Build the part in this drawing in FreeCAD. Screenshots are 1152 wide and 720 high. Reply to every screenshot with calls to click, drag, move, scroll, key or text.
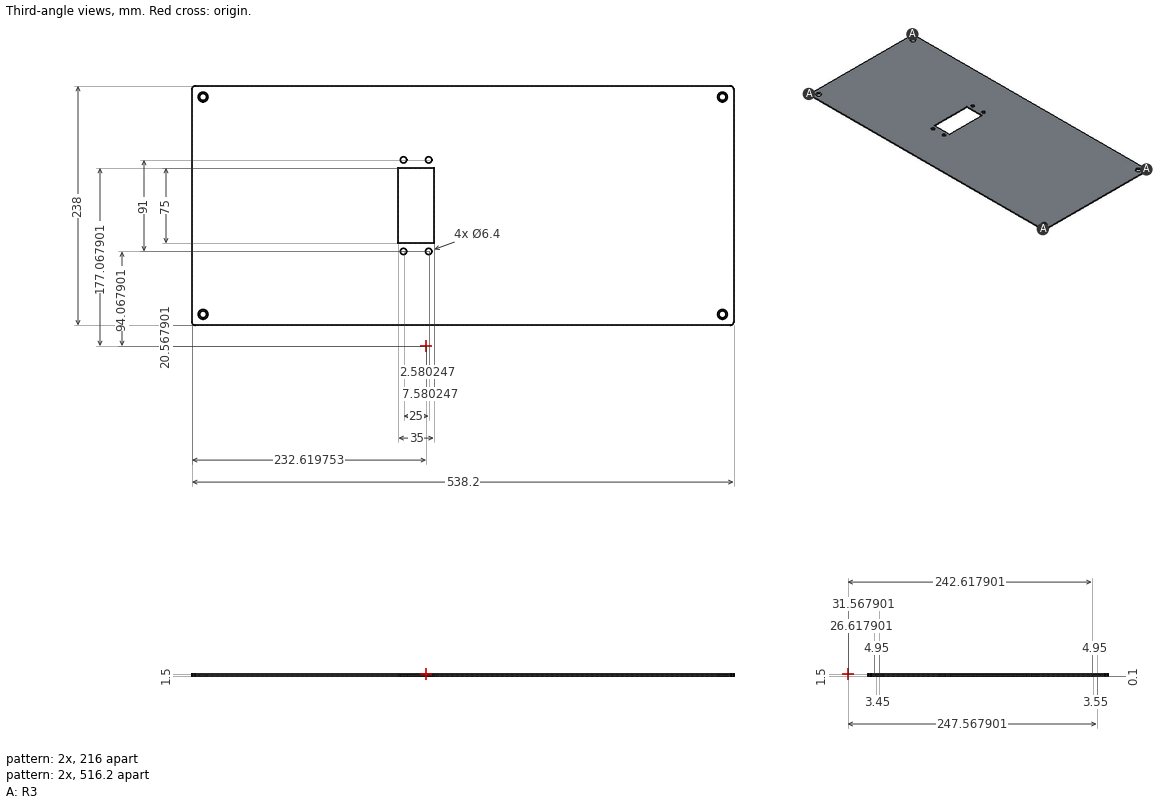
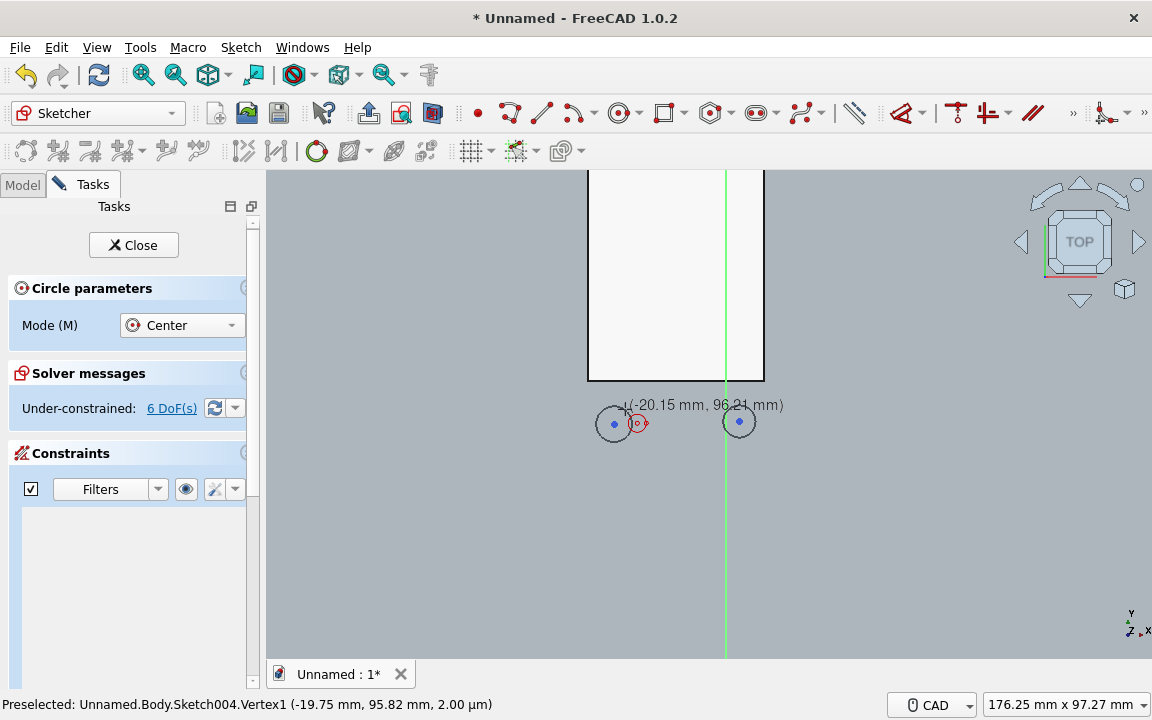
scroll(625, 412, down, 6)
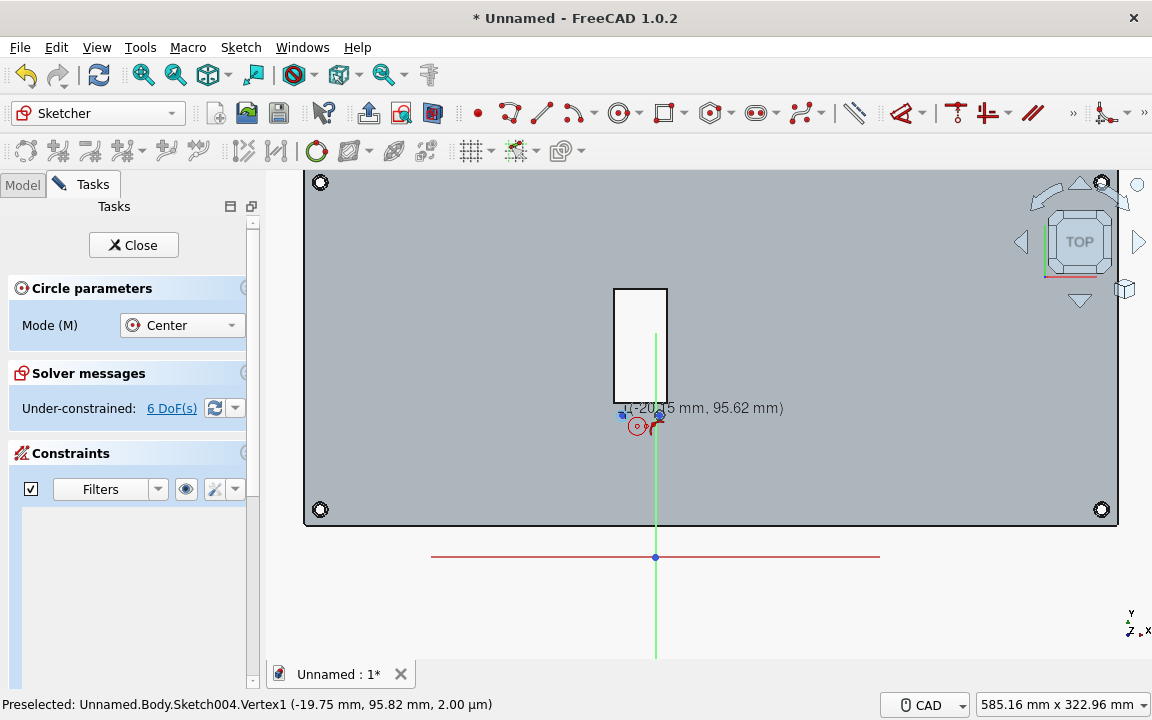
scroll(660, 277, up, 8)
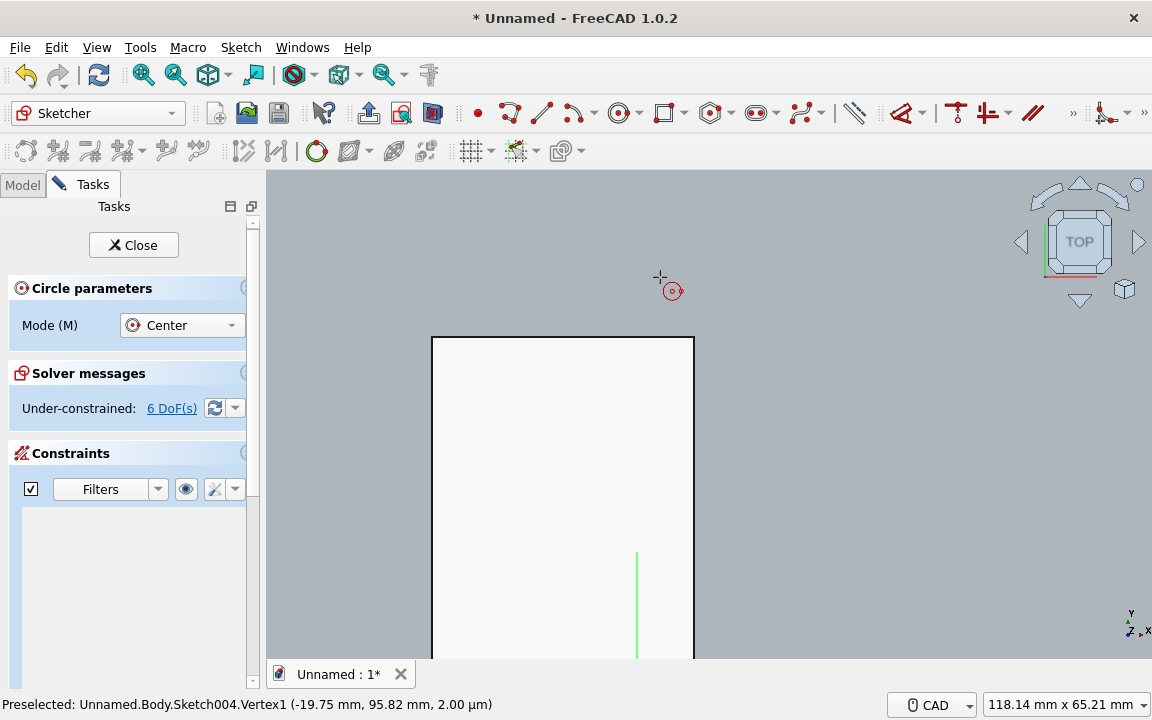
click(657, 277)
click(674, 260)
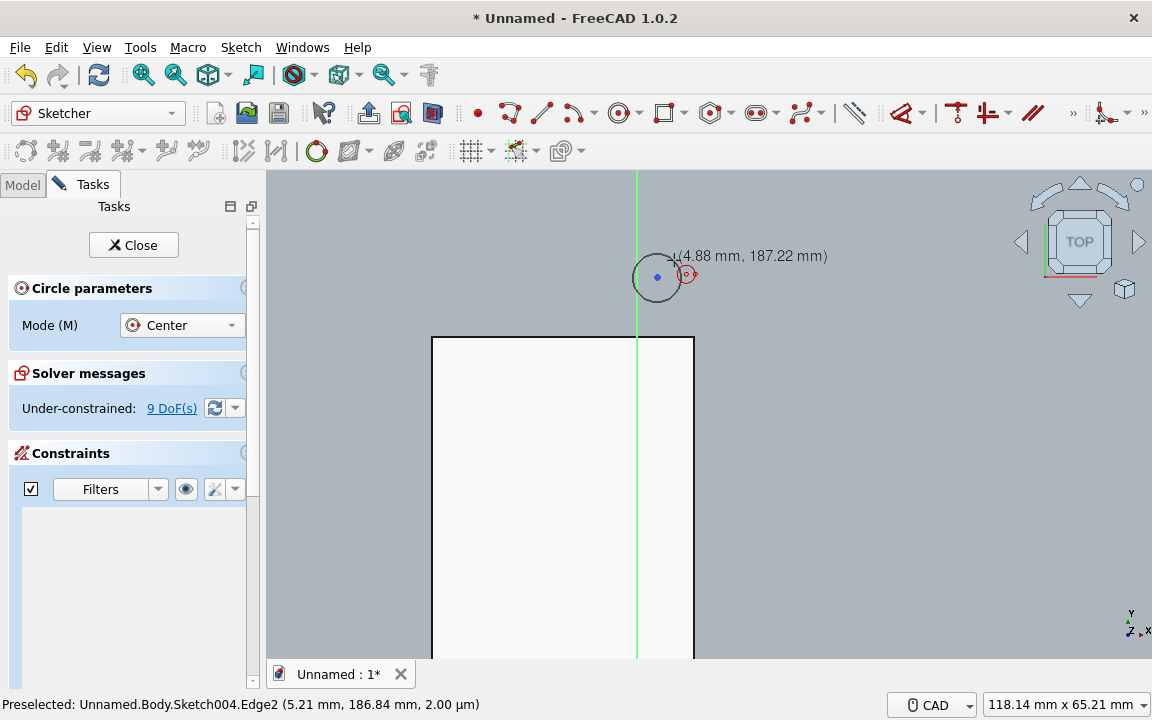
scroll(660, 277, down, 8)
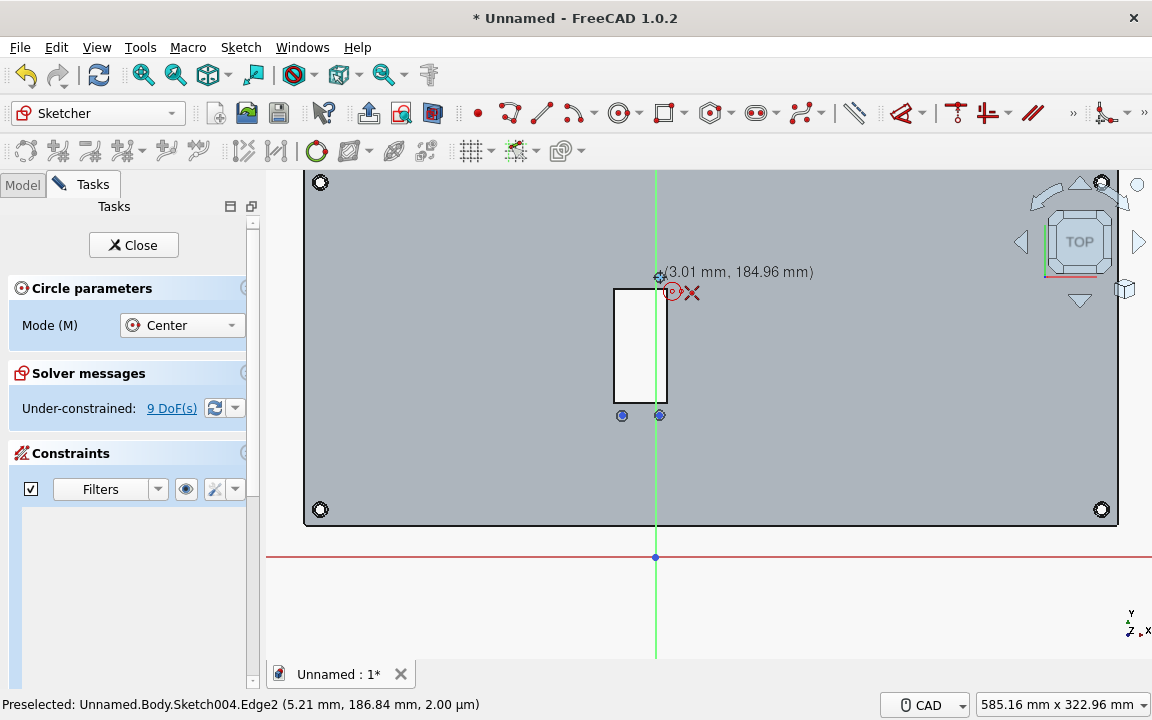
click(622, 277)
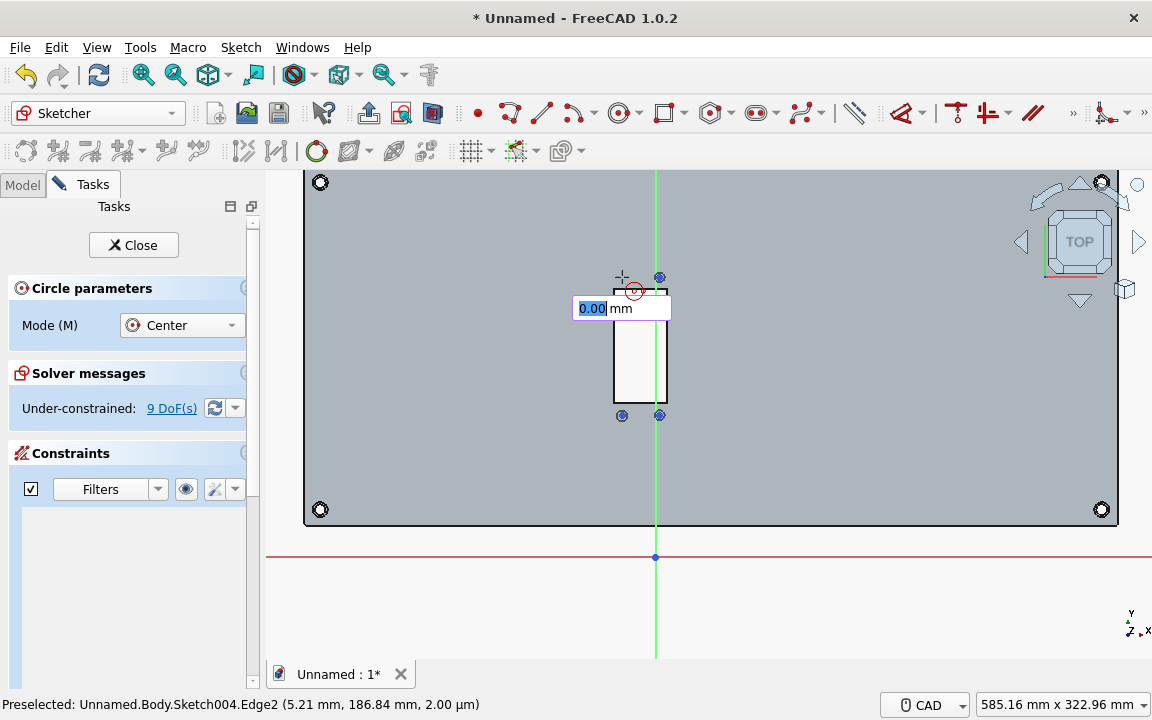
scroll(625, 274, up, 6)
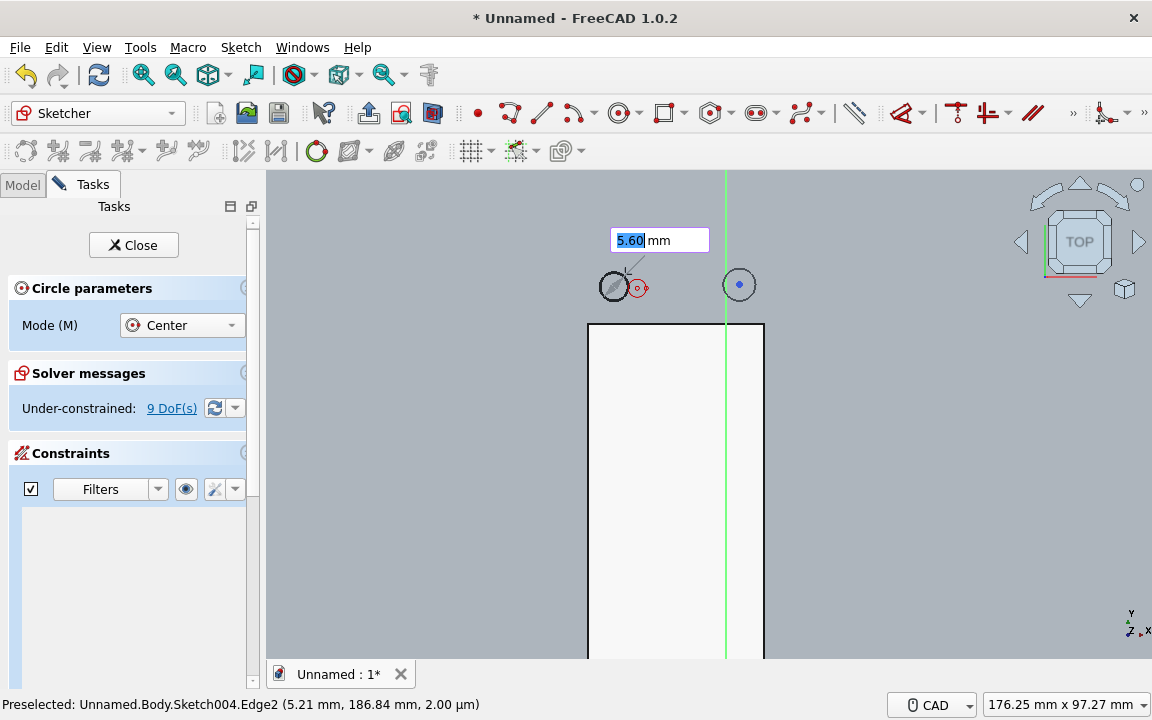
click(625, 273)
key(Escape)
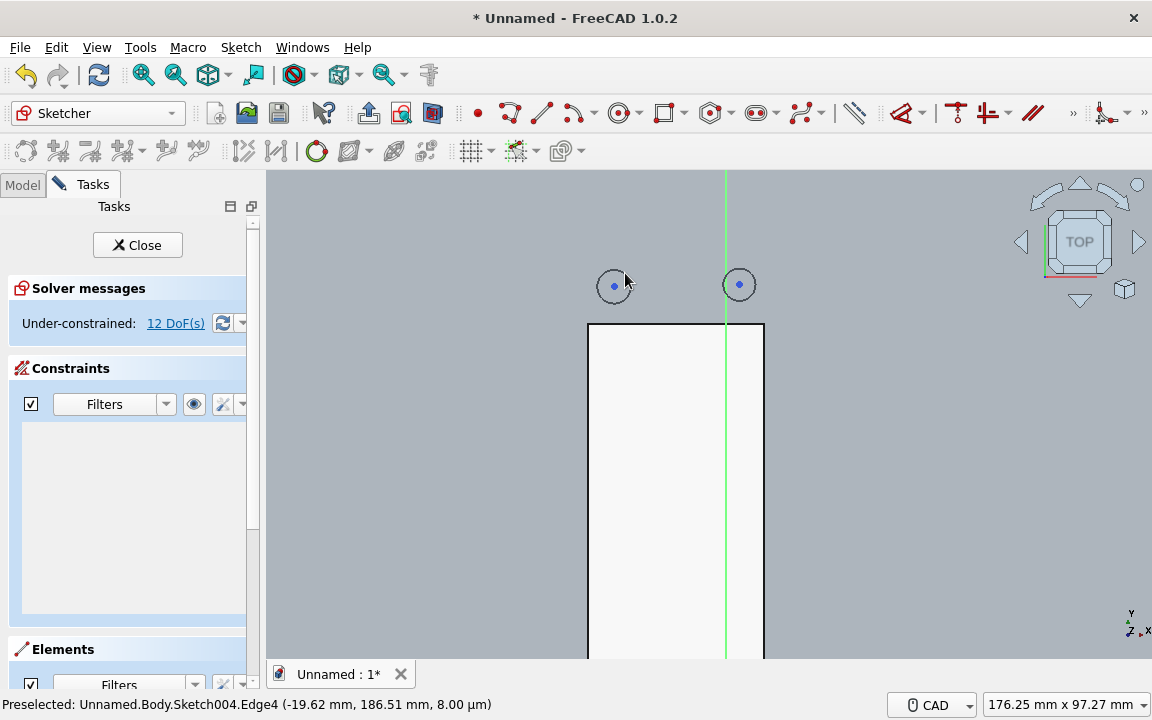
scroll(625, 274, down, 6)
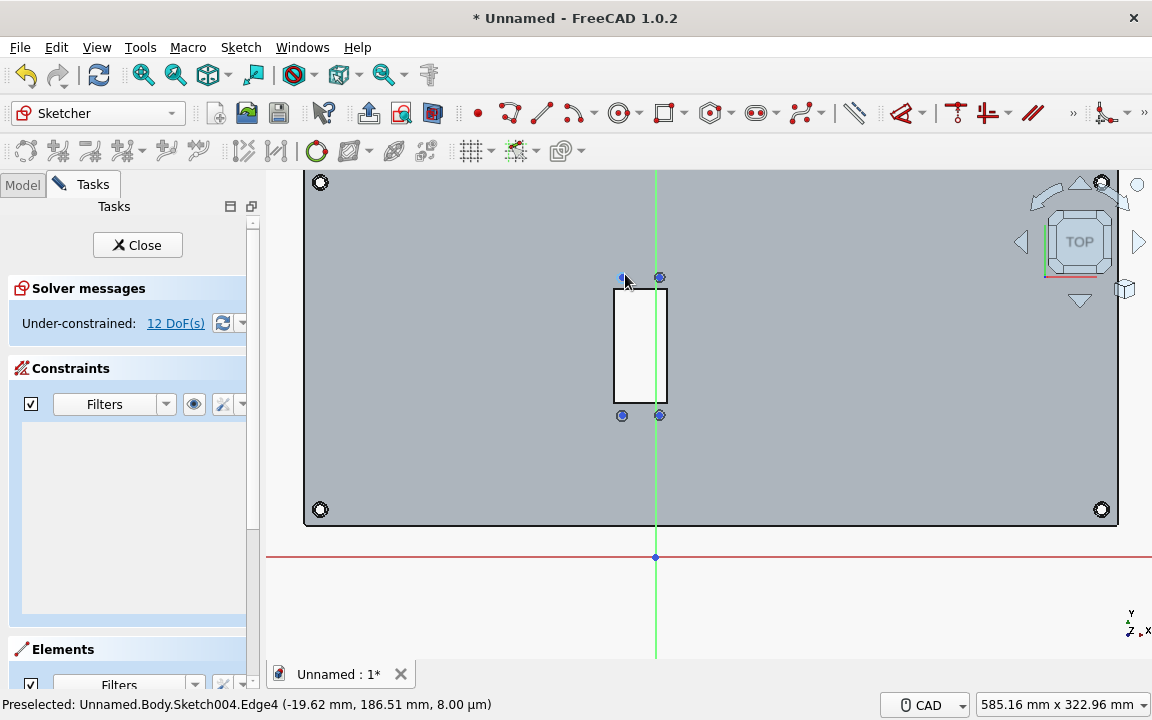
scroll(663, 412, up, 6)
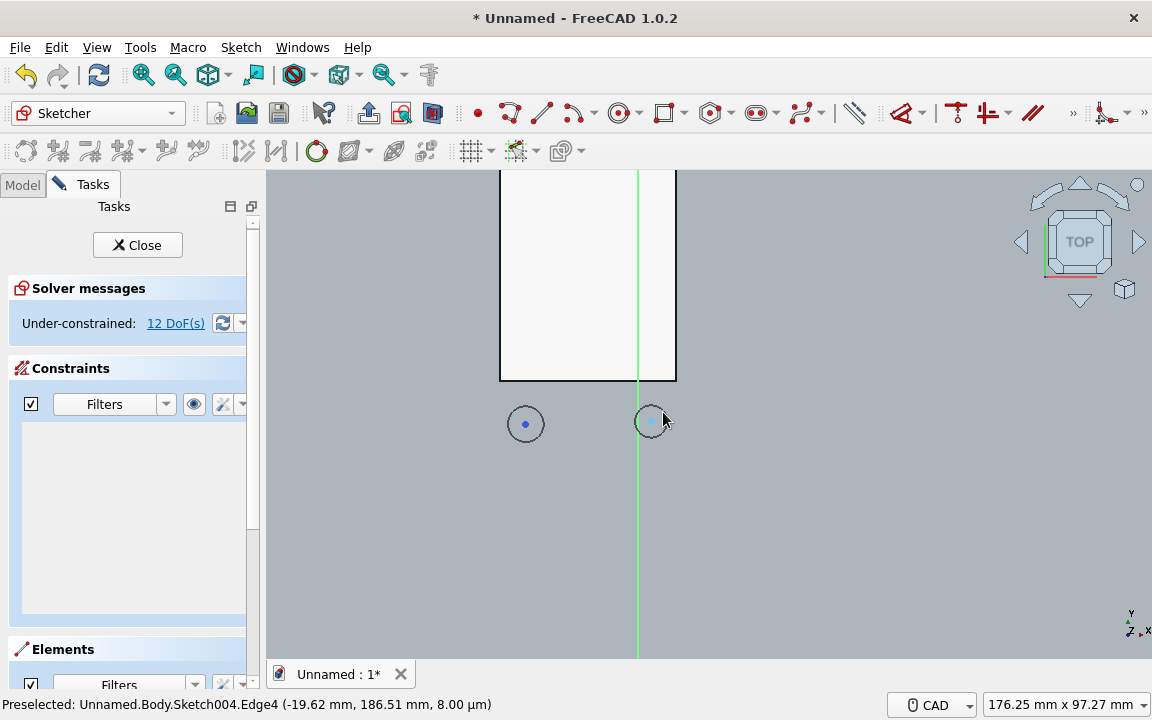
click(663, 410)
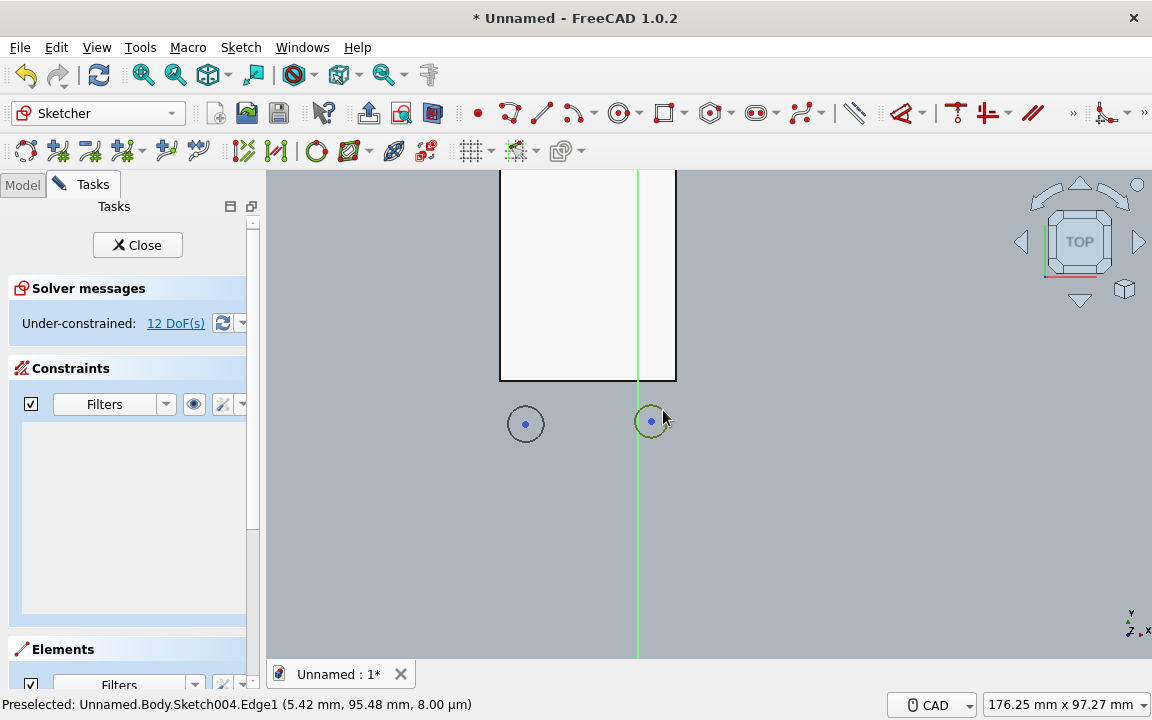
click(538, 411)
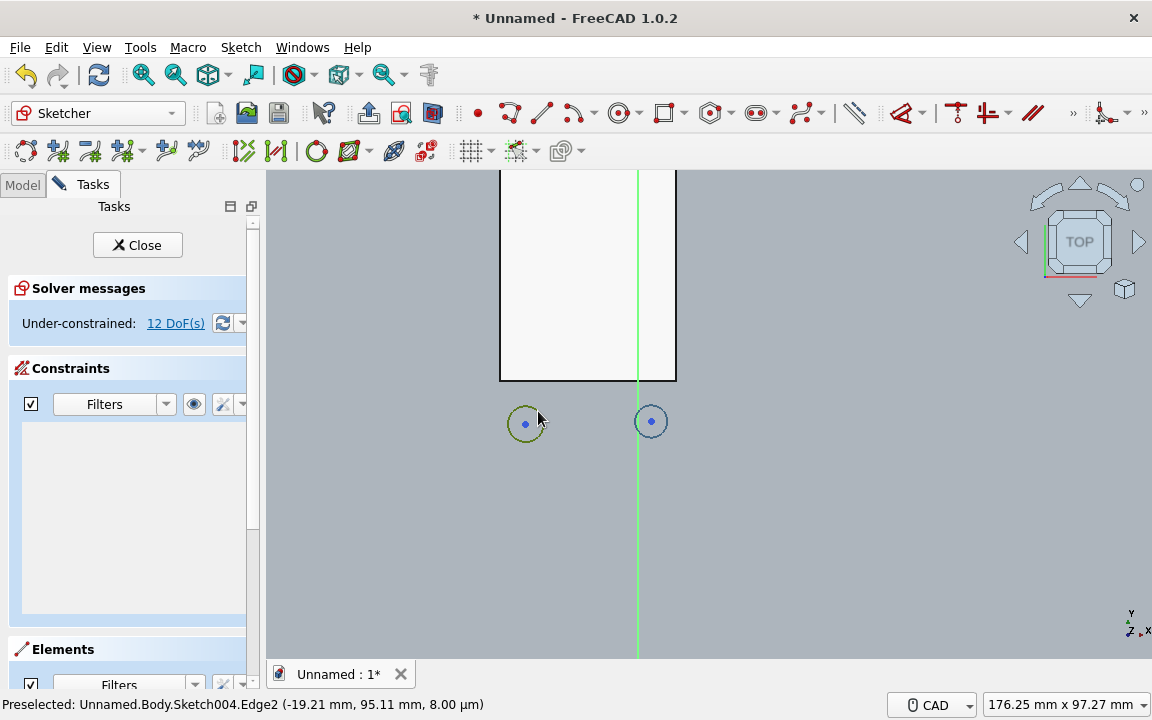
scroll(663, 412, down, 6)